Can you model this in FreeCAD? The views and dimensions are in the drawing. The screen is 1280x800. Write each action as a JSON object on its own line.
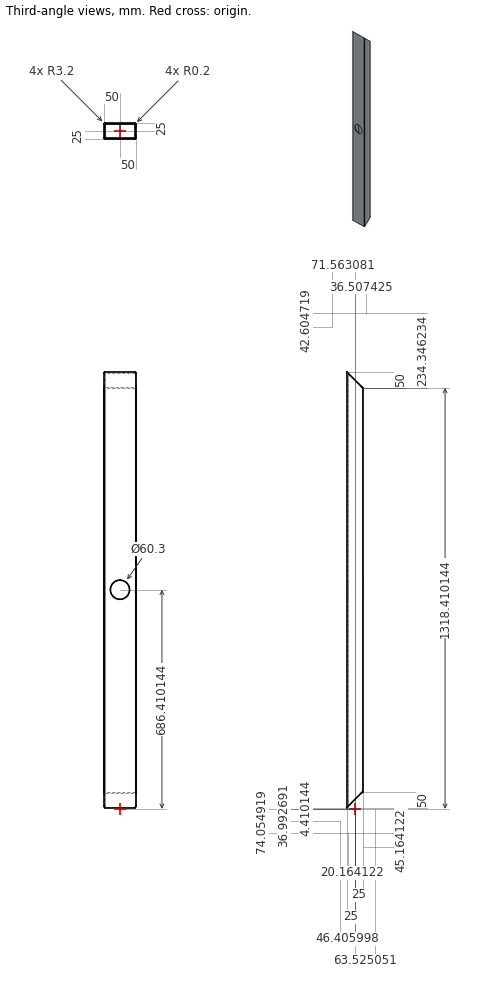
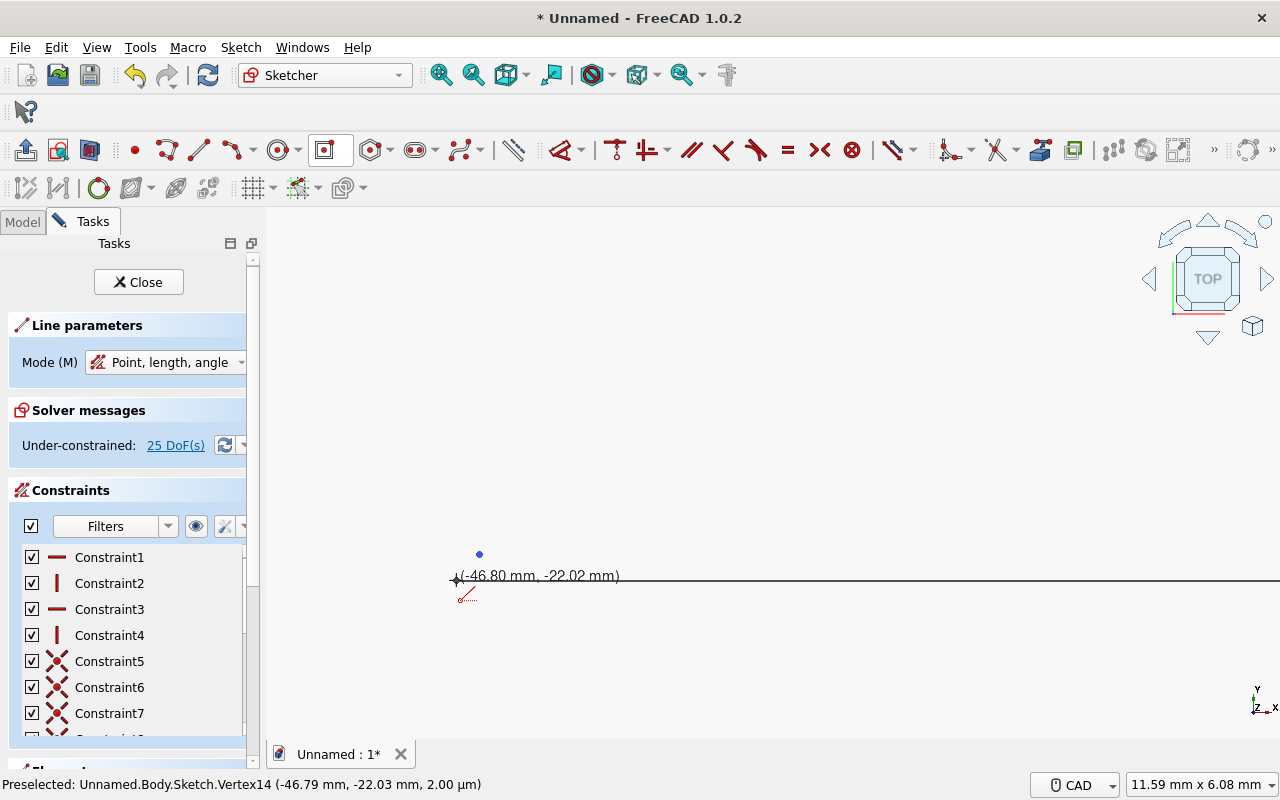
{"action": "left_click", "coordinate": [438, 562]}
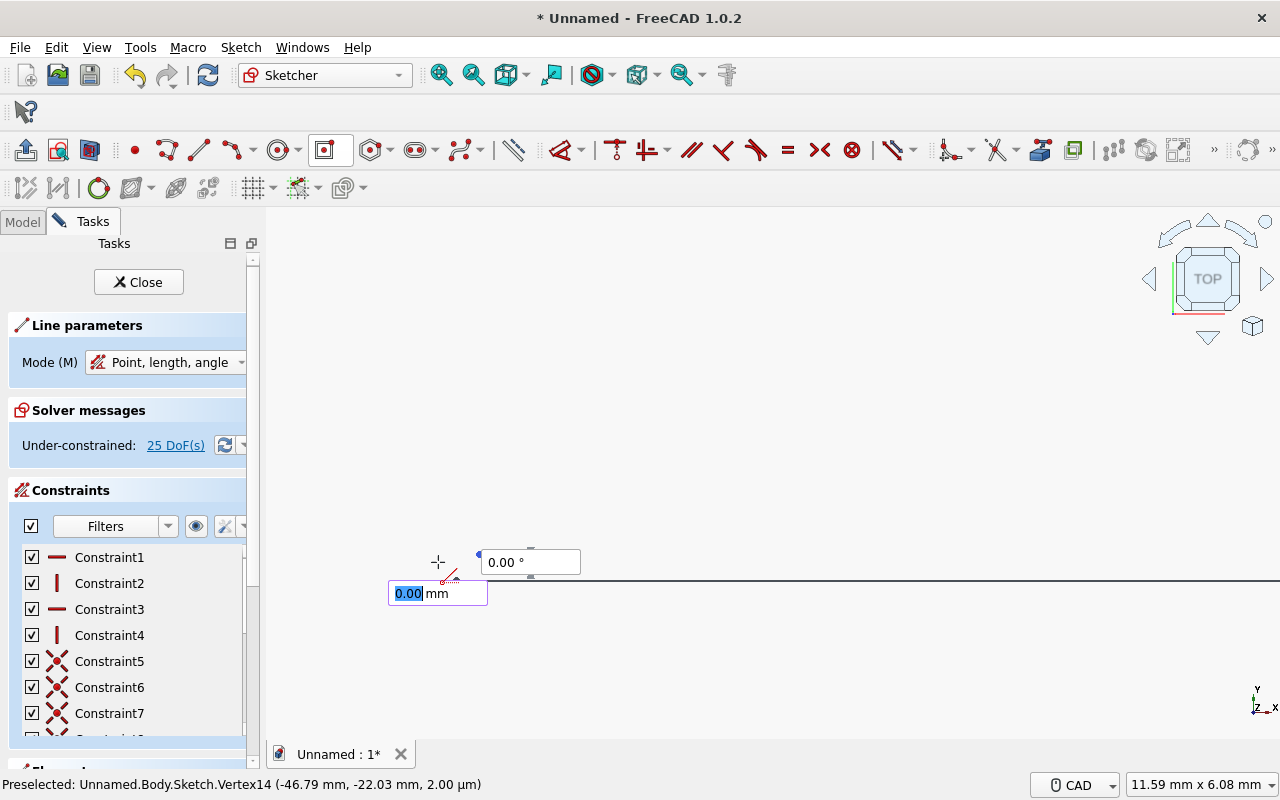
{"action": "scroll", "coordinate": [455, 591], "scroll_direction": "down", "scroll_amount": 14}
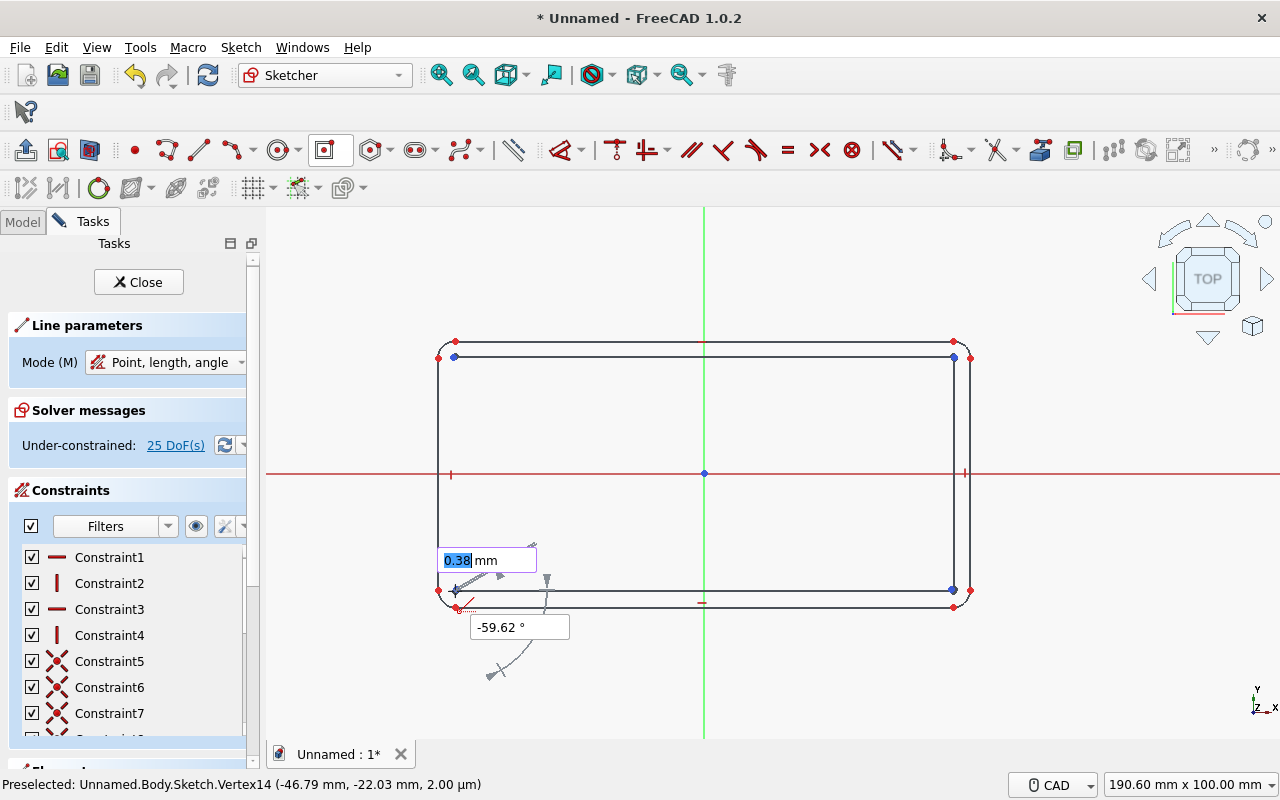
{"action": "scroll", "coordinate": [454, 358], "scroll_direction": "up", "scroll_amount": 14}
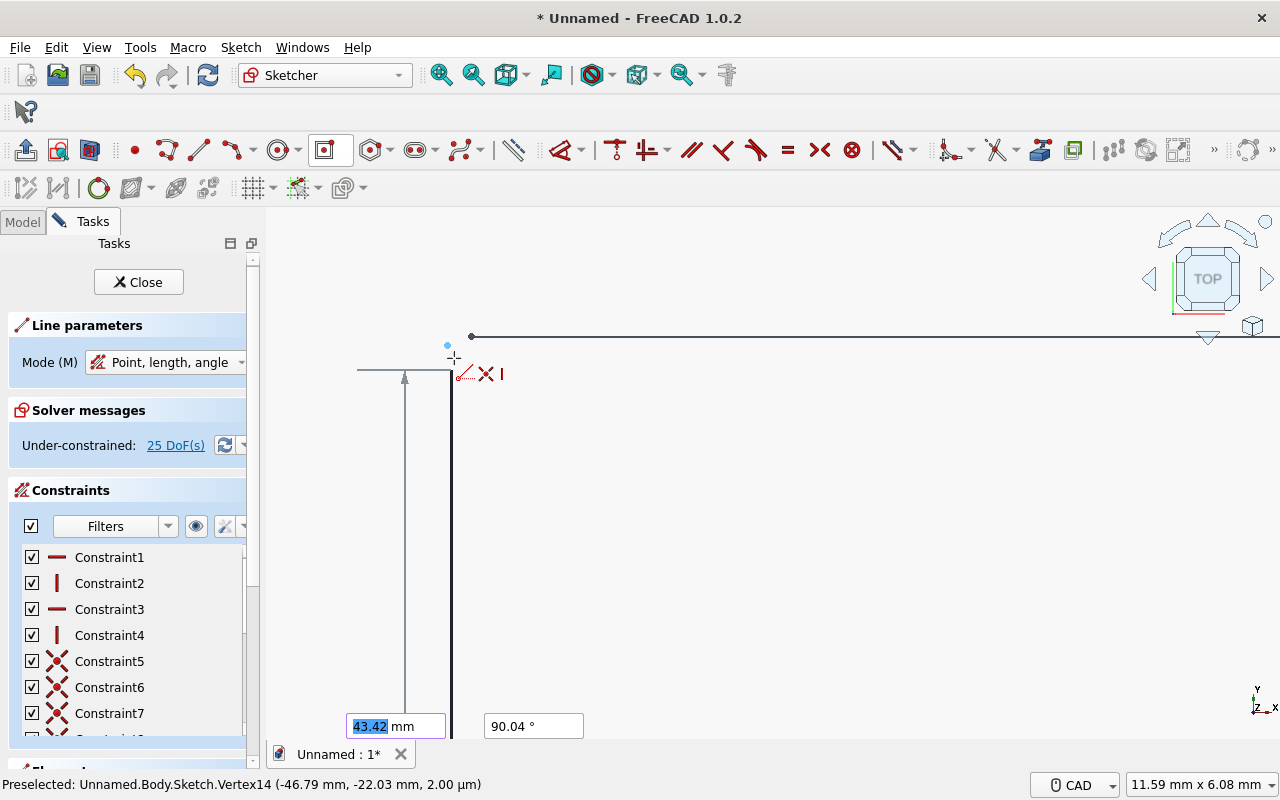
{"action": "left_click", "coordinate": [453, 353]}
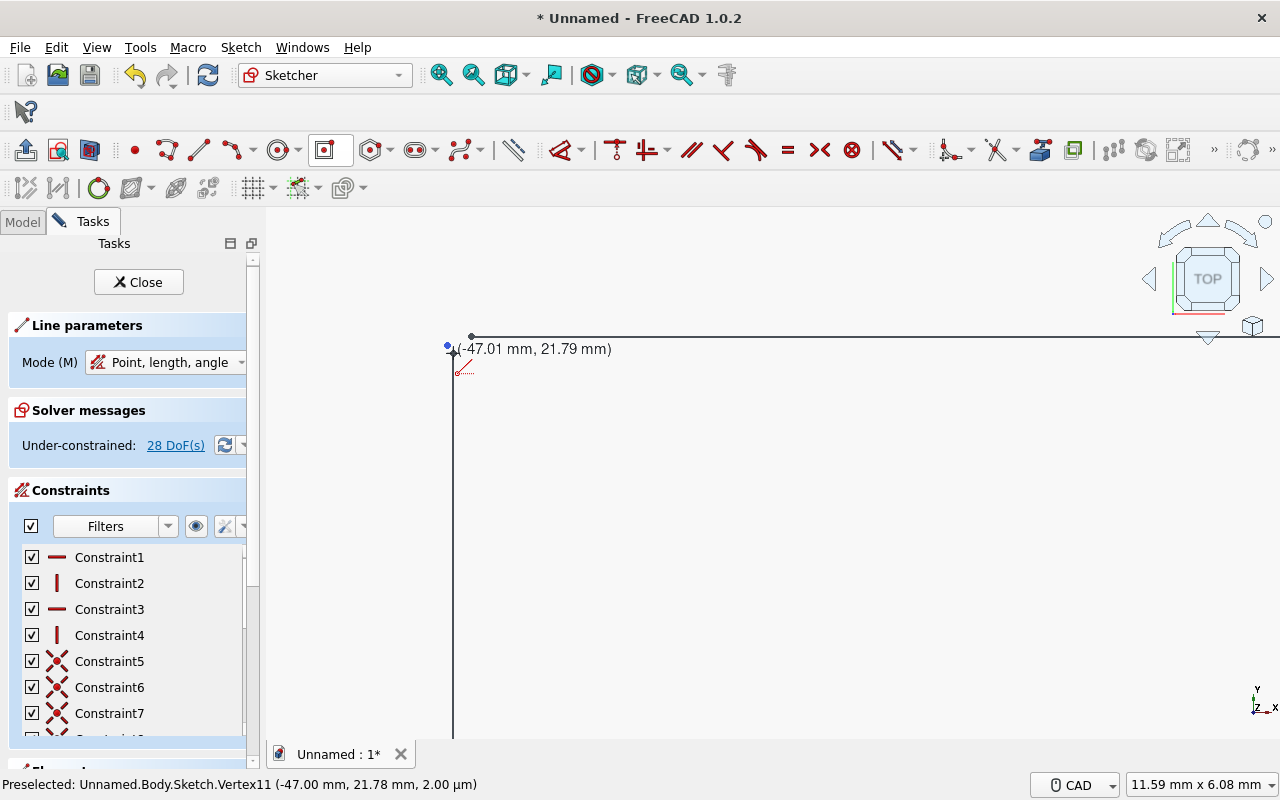
{"action": "left_click", "coordinate": [232, 150]}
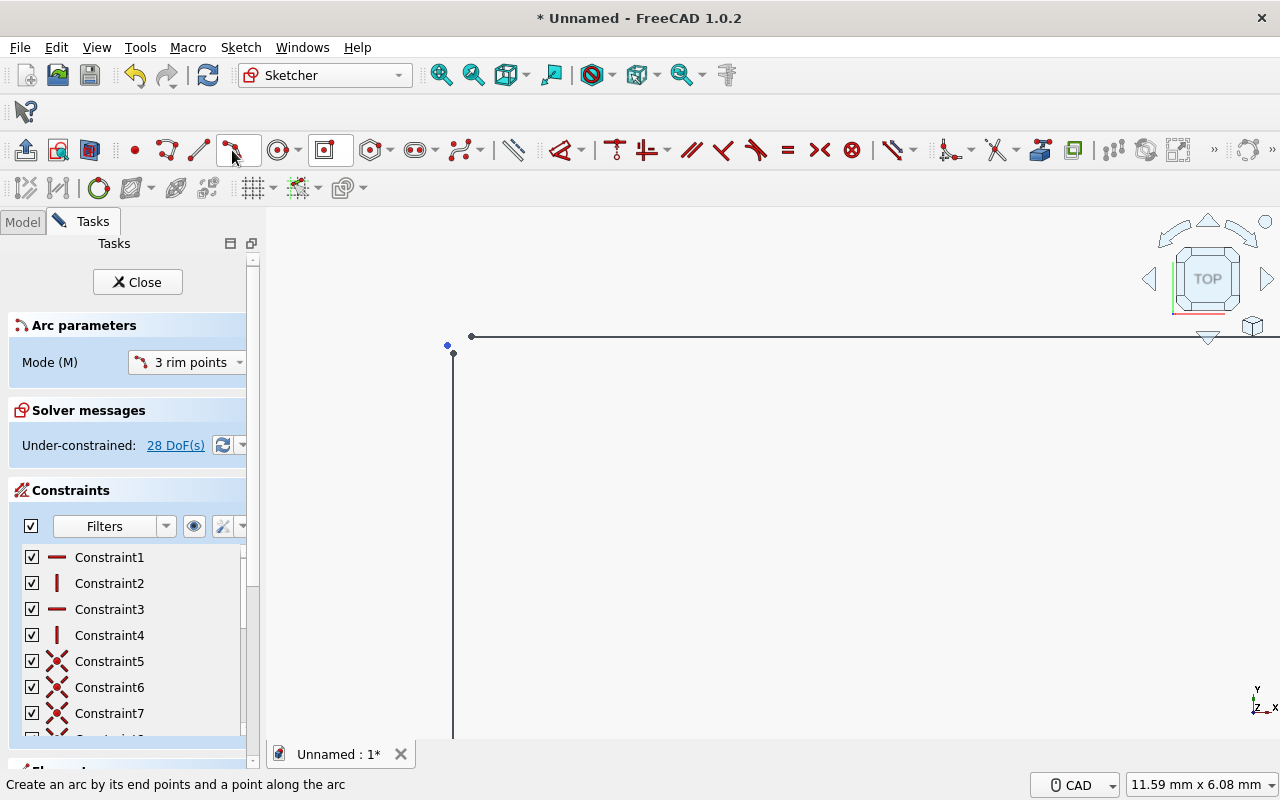
{"action": "scroll", "coordinate": [454, 357], "scroll_direction": "down", "scroll_amount": 14}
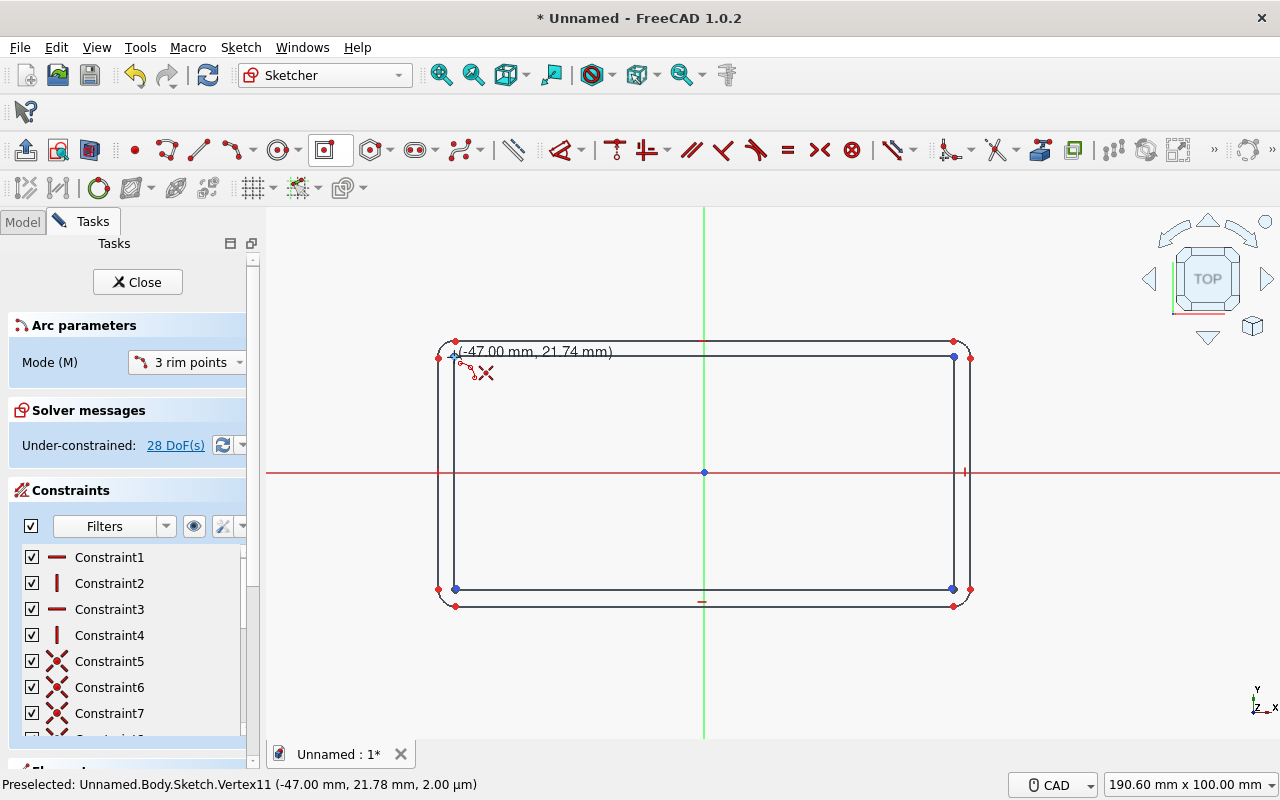
{"action": "scroll", "coordinate": [953, 356], "scroll_direction": "up", "scroll_amount": 14}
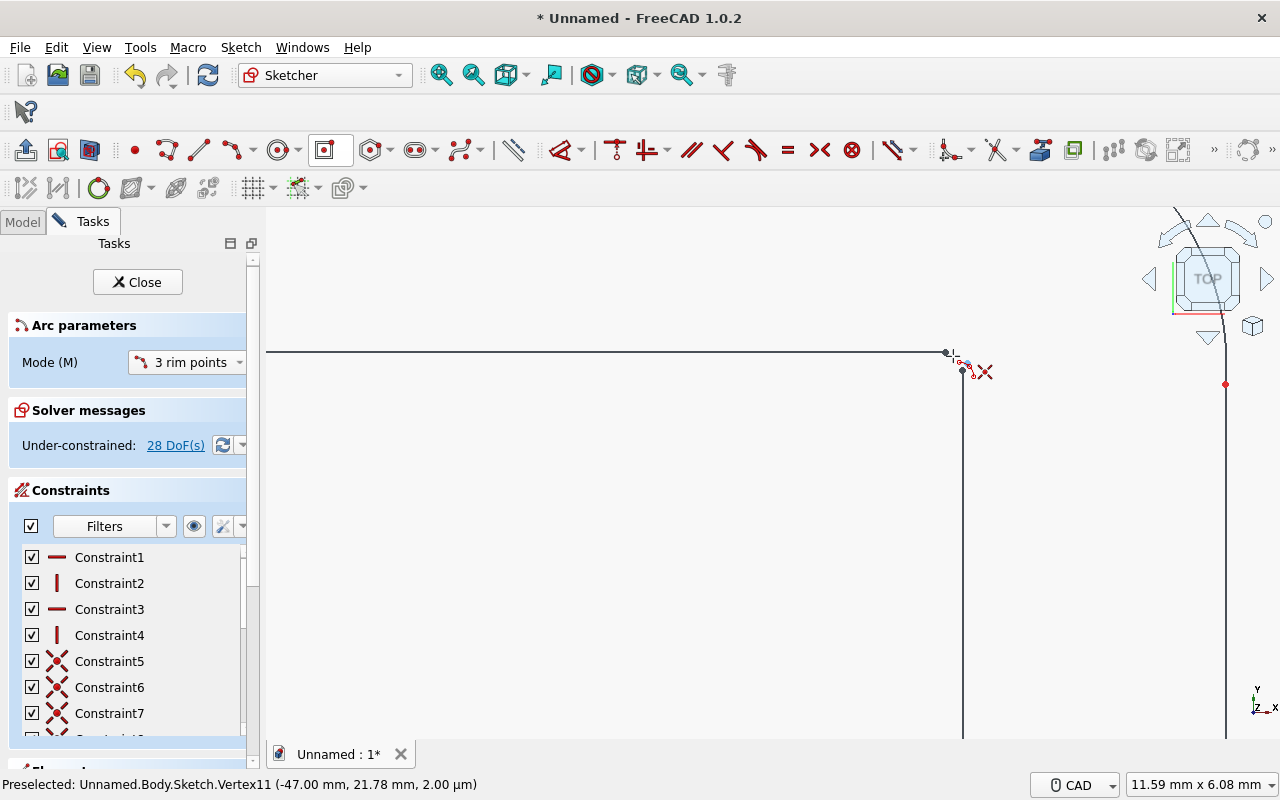
{"action": "left_click", "coordinate": [946, 352]}
{"action": "left_click", "coordinate": [963, 370]}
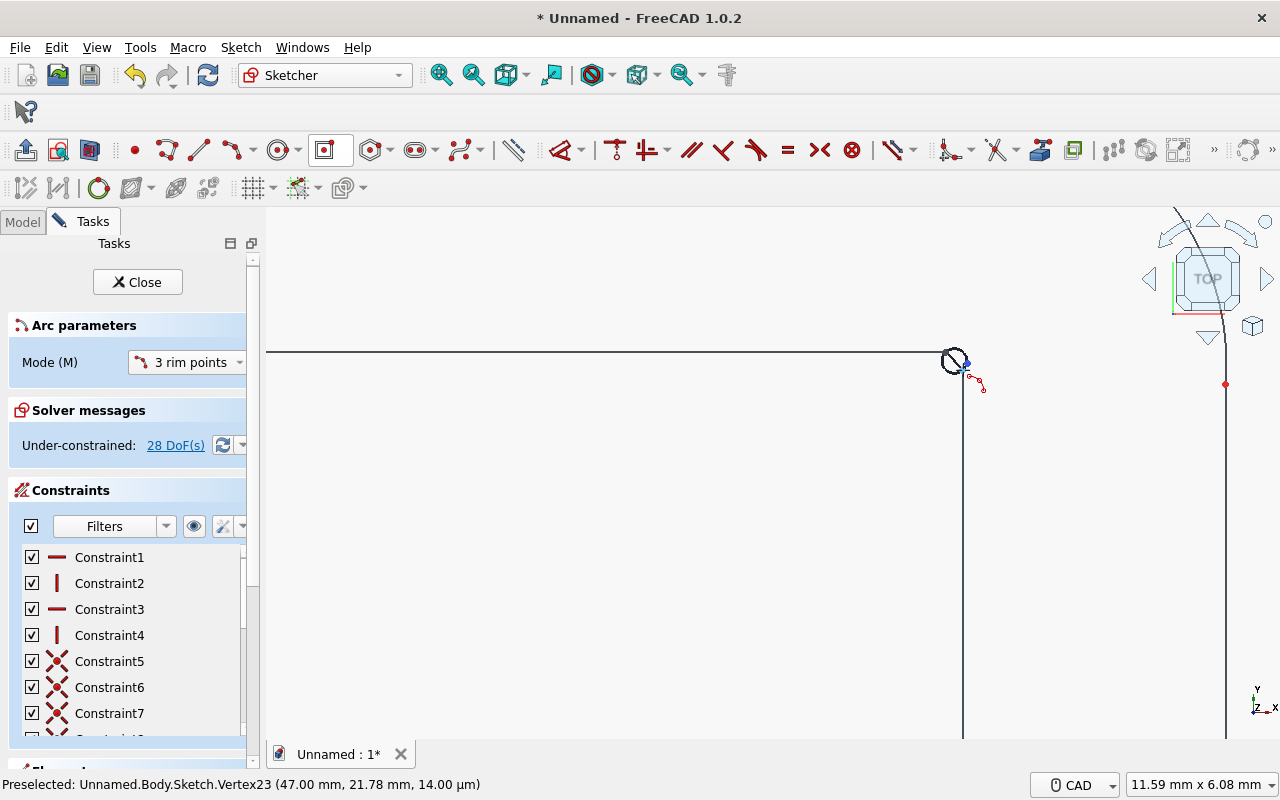
{"action": "scroll", "coordinate": [958, 356], "scroll_direction": "up", "scroll_amount": 6}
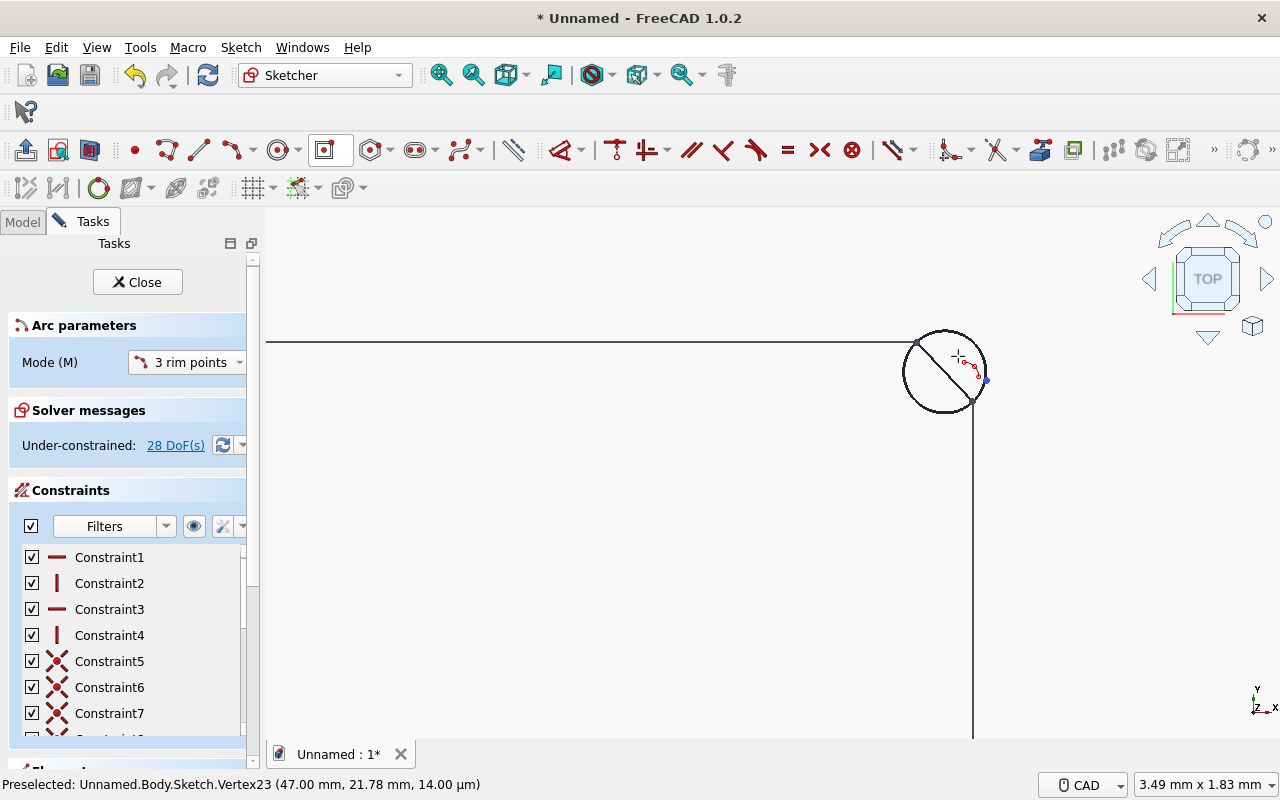
{"action": "left_click", "coordinate": [956, 356]}